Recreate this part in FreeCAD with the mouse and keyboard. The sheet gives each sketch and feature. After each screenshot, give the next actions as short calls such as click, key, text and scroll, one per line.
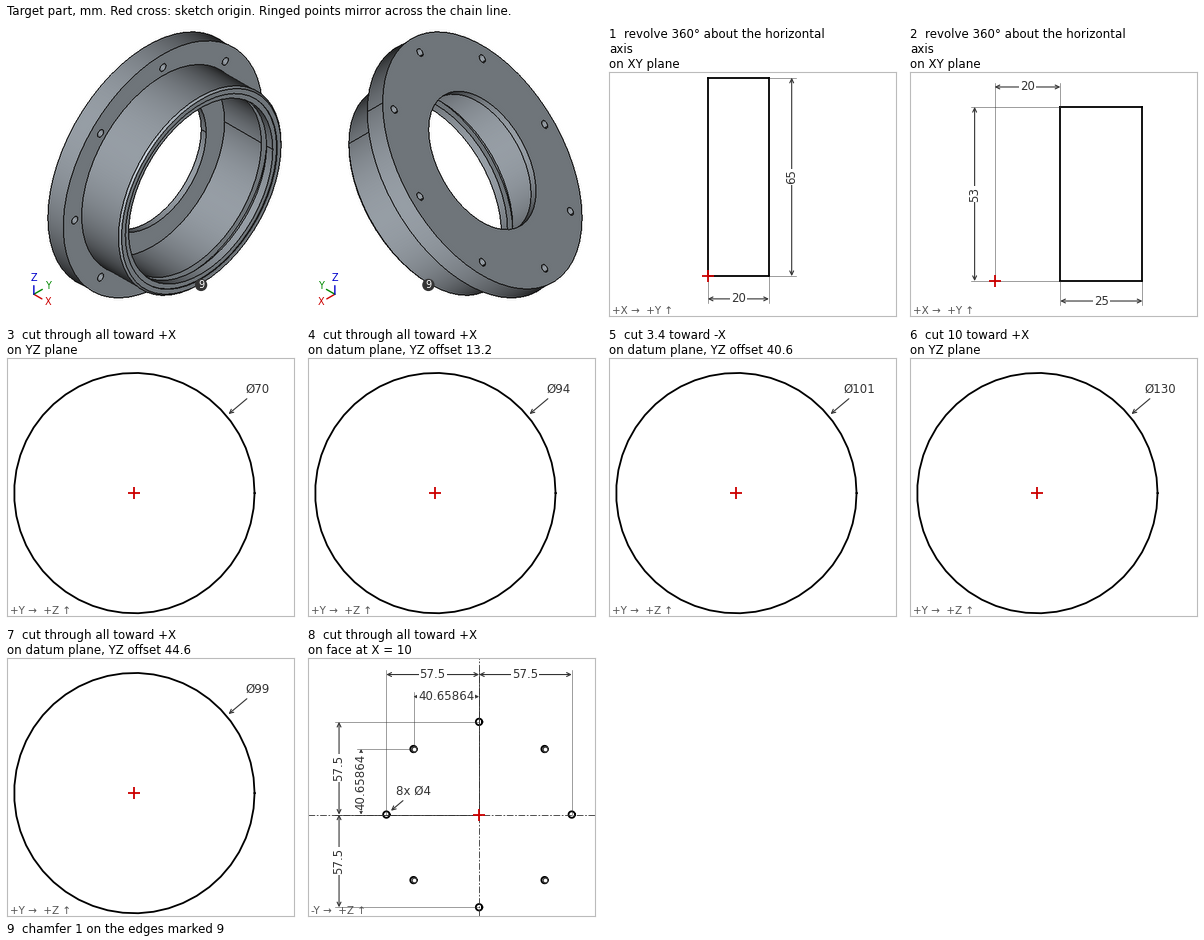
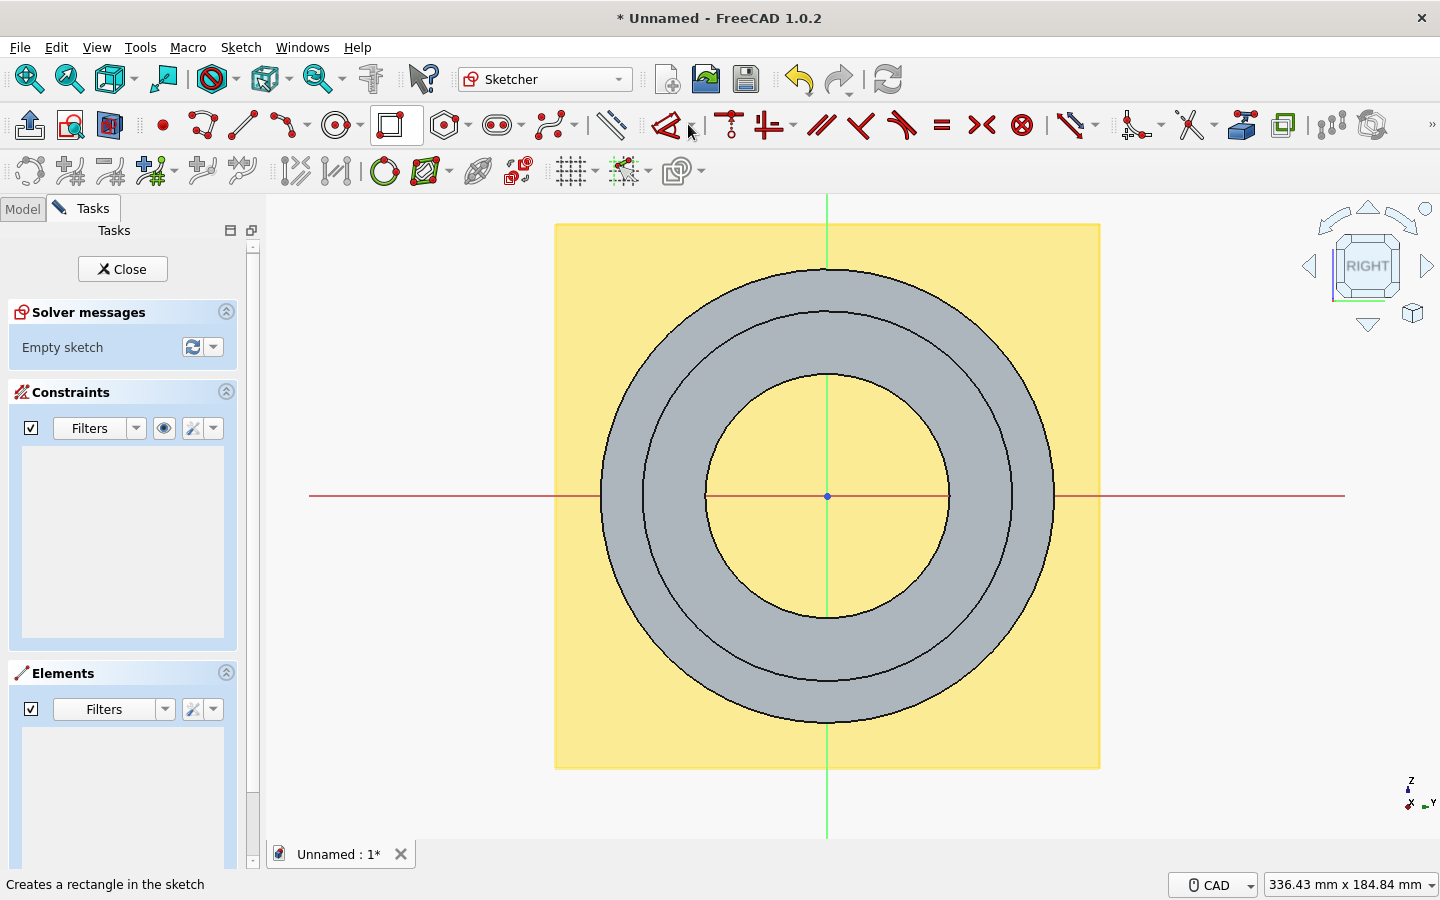
click(110, 126)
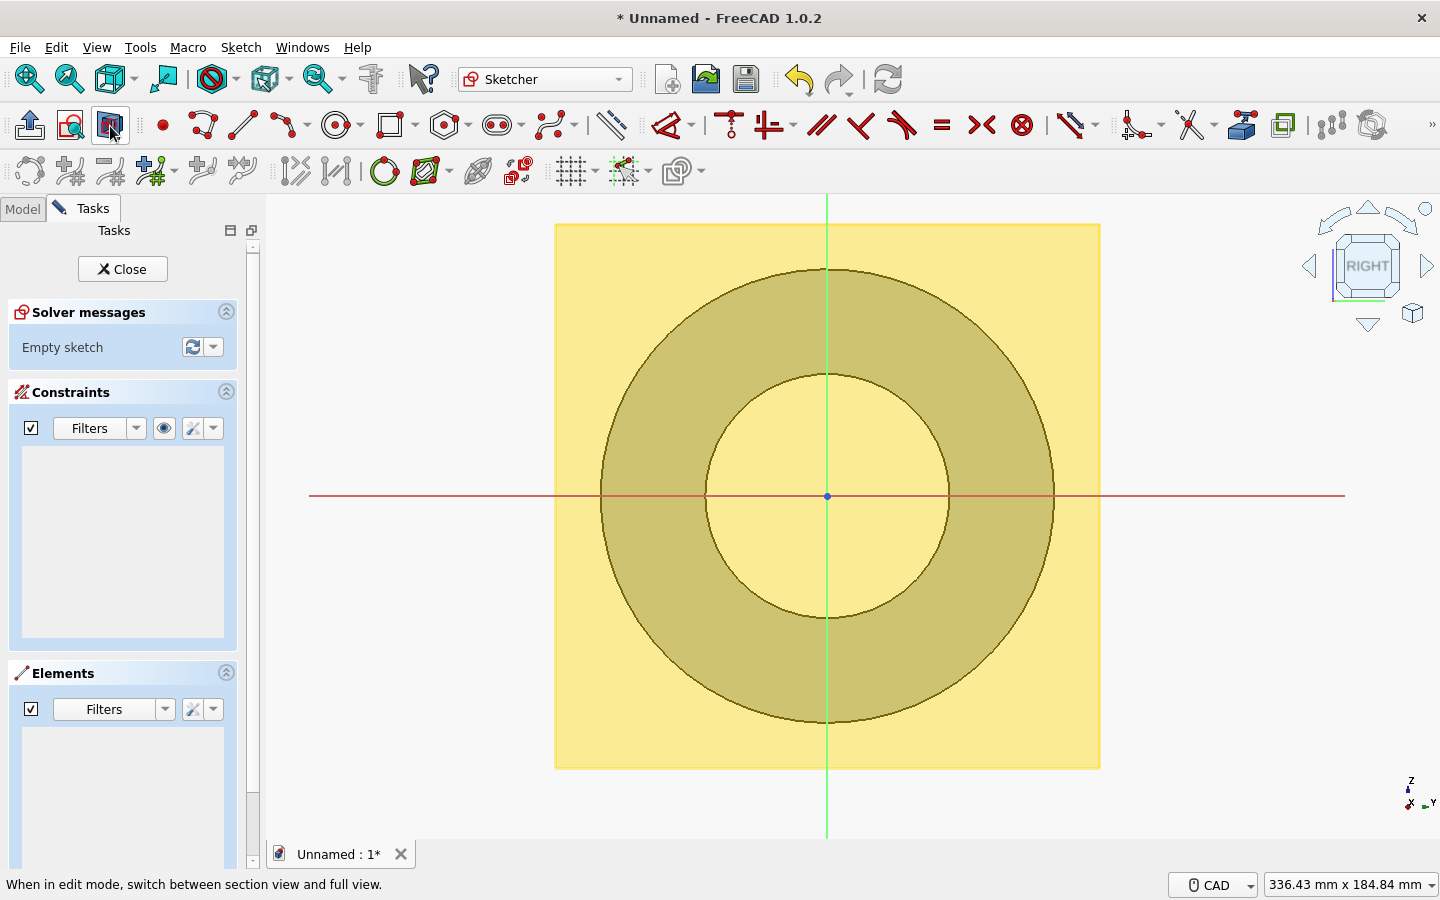
click(336, 126)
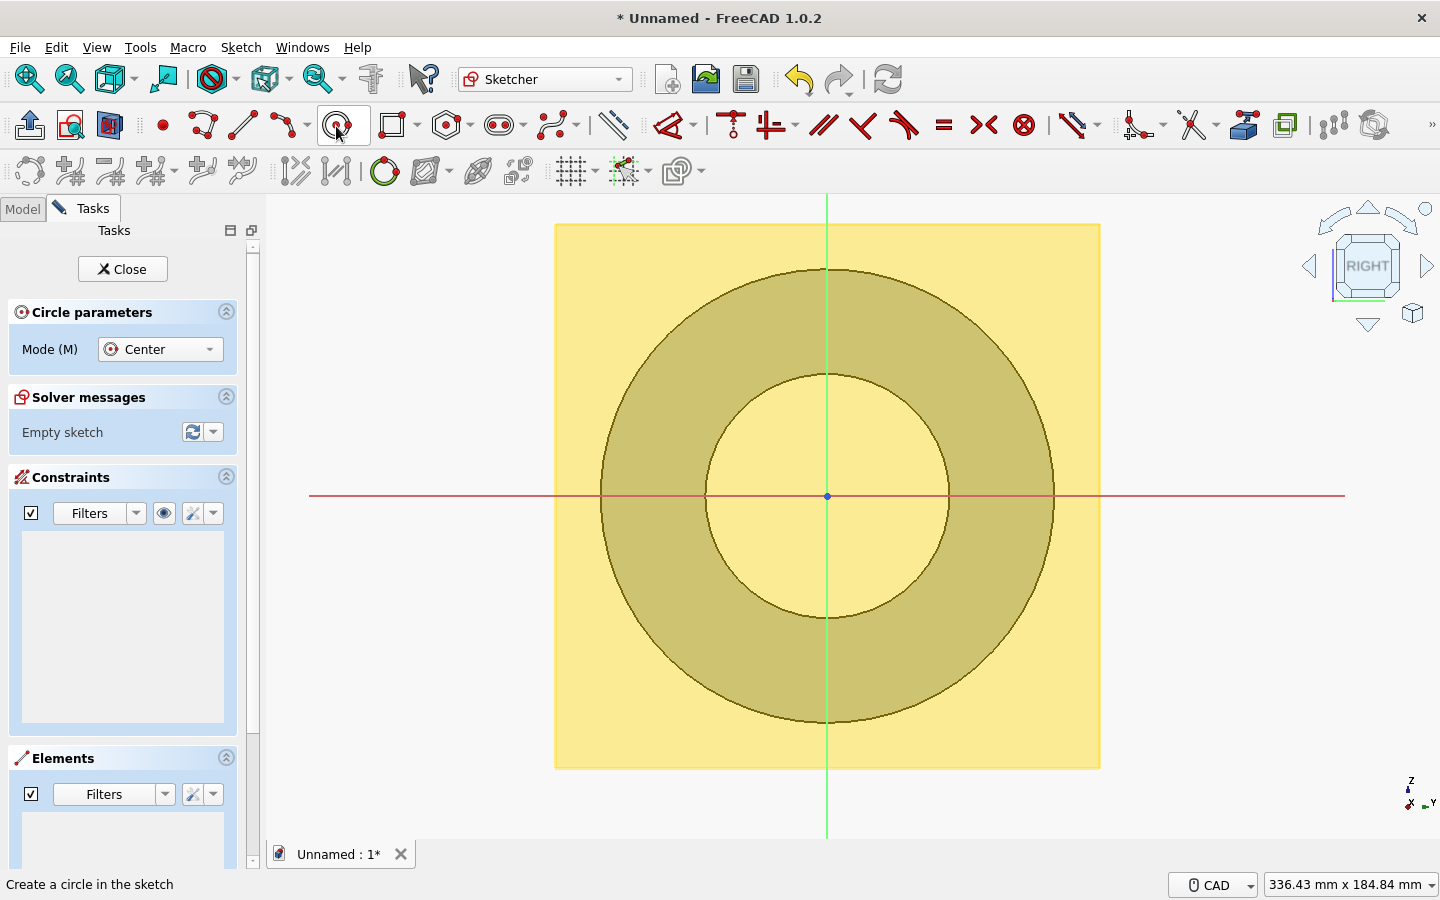
click(827, 496)
click(943, 380)
key(Escape)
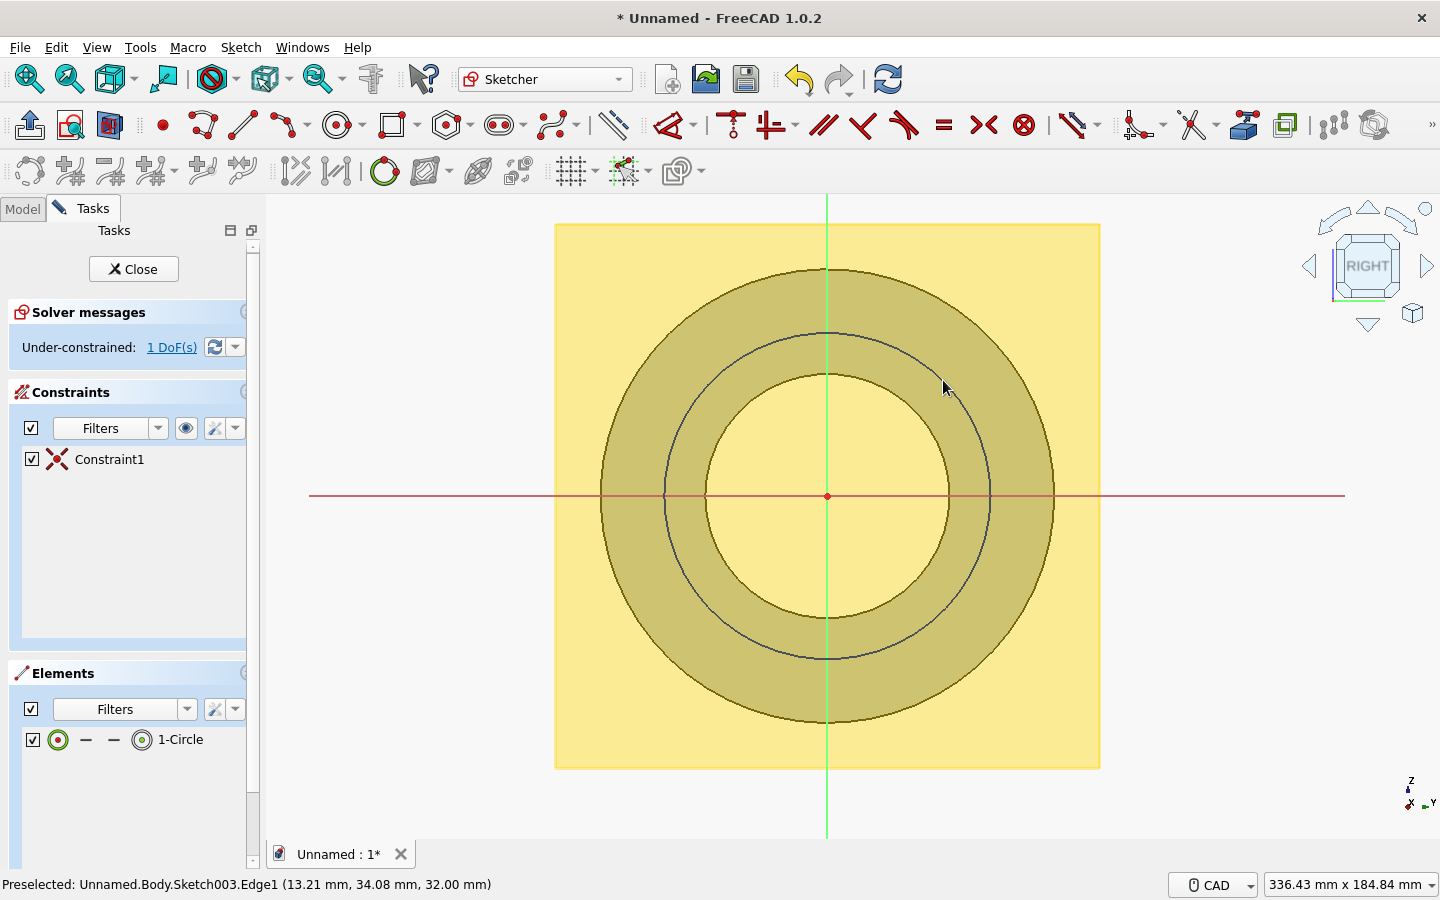
click(668, 126)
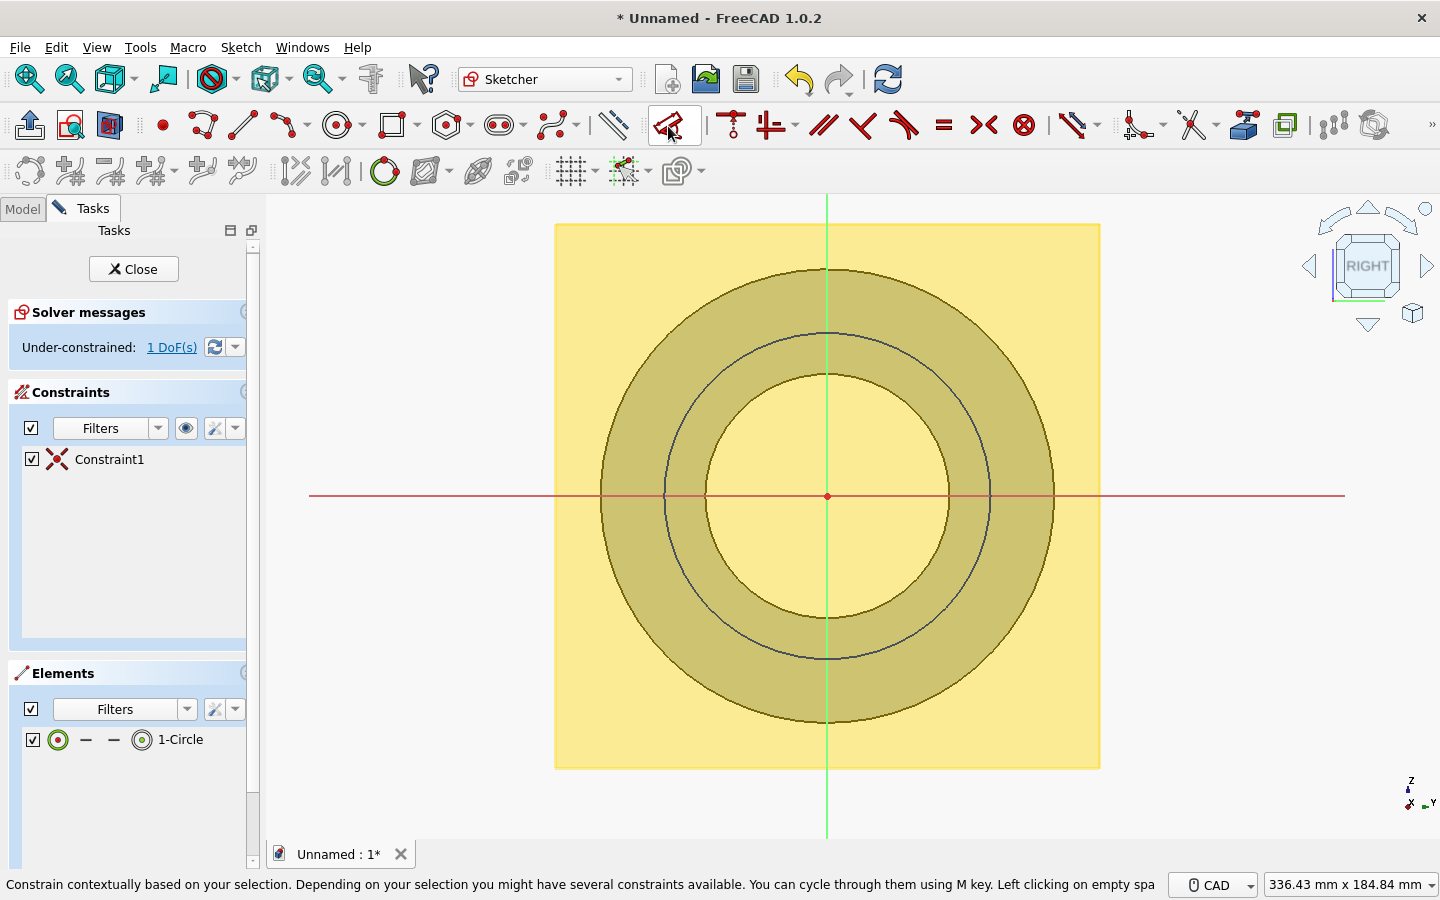
click(942, 380)
click(964, 357)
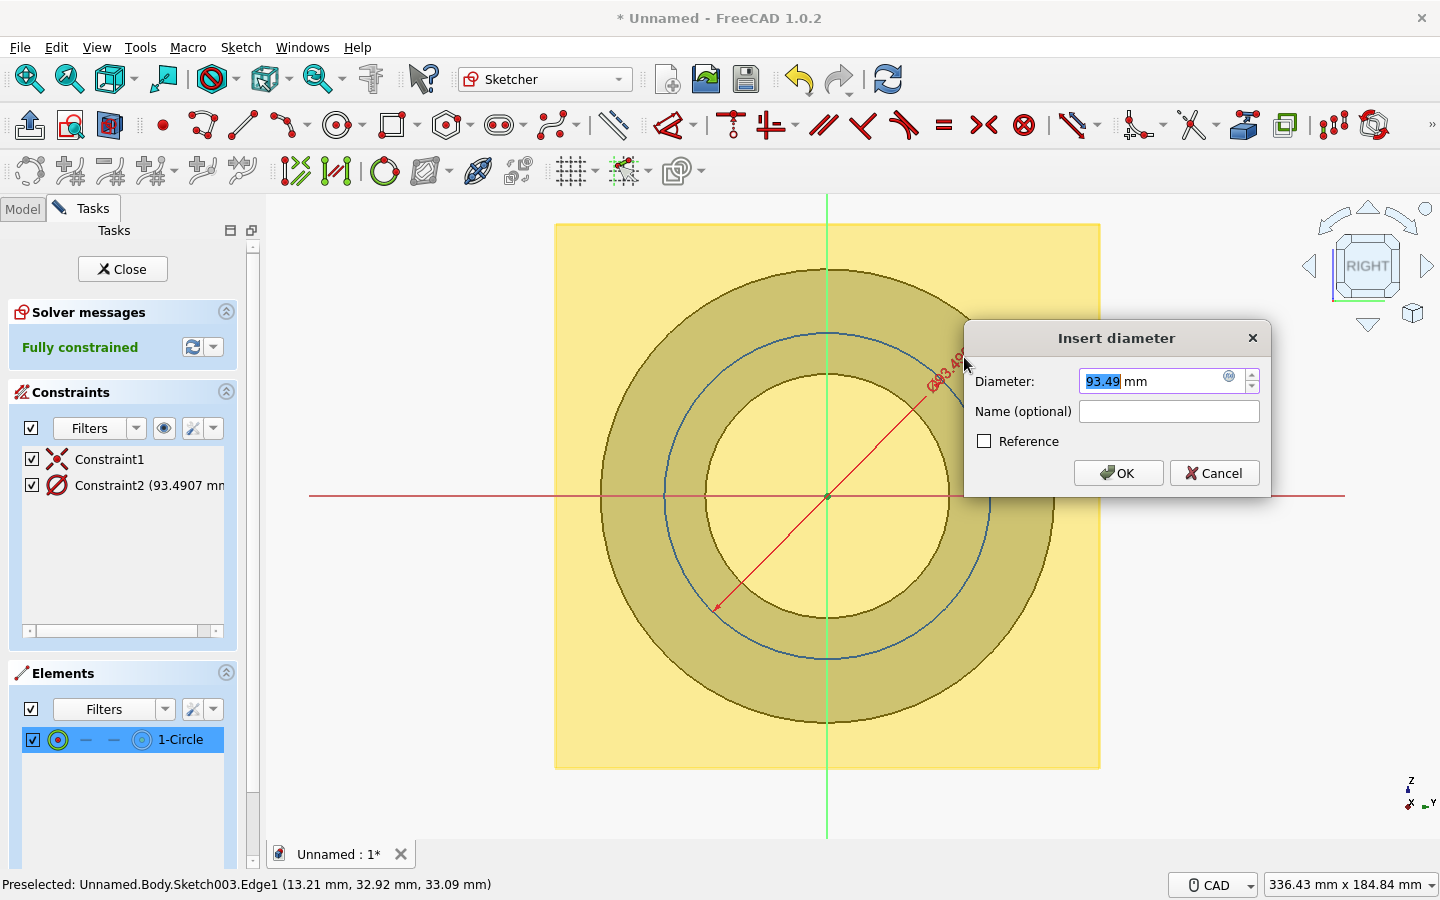
text(94)
key(Return)
key(Escape)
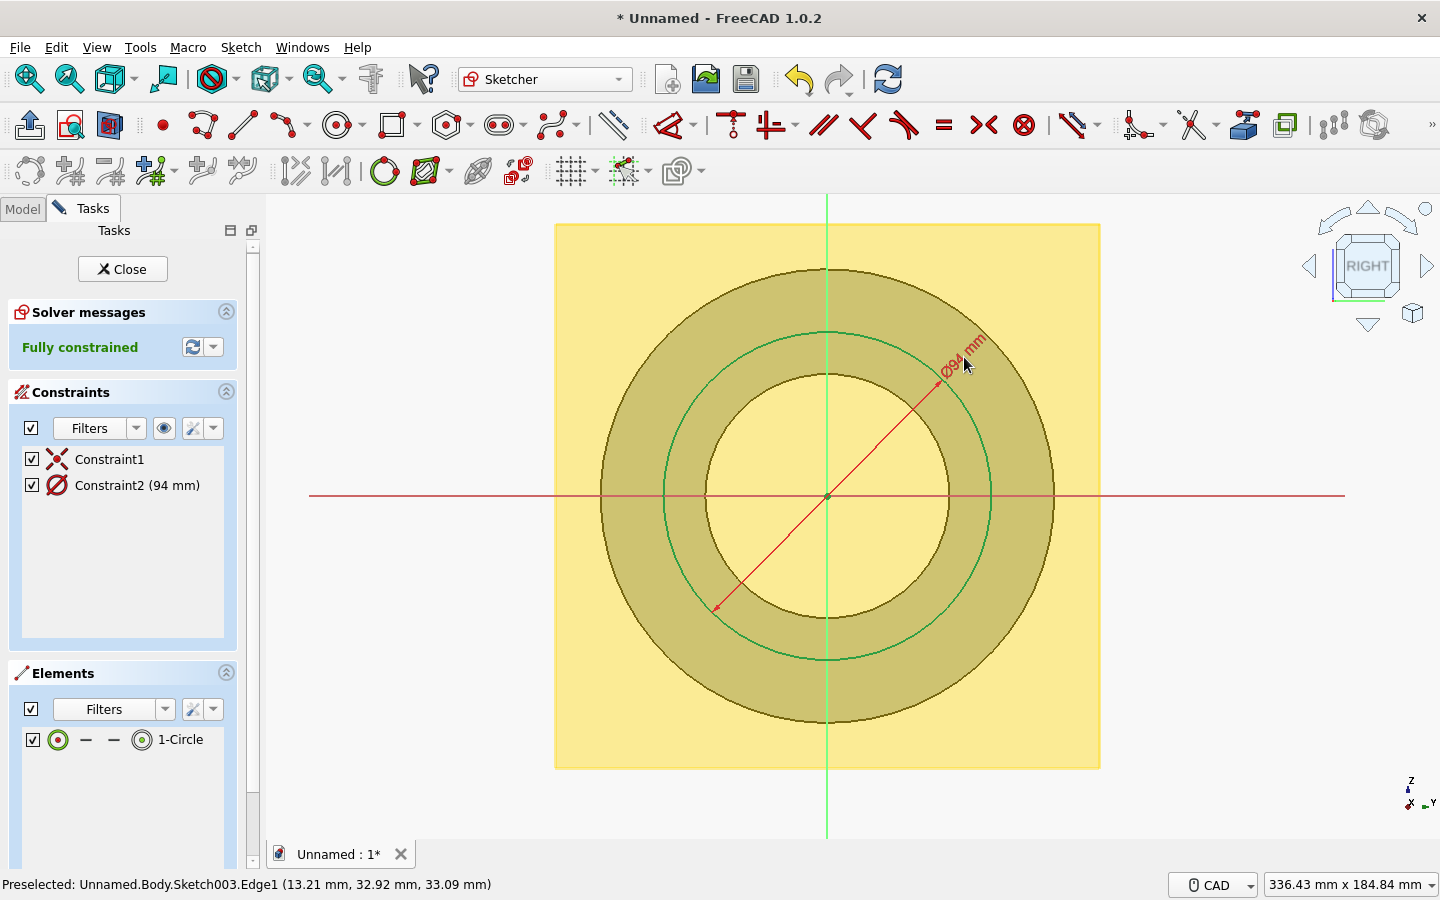
click(123, 269)